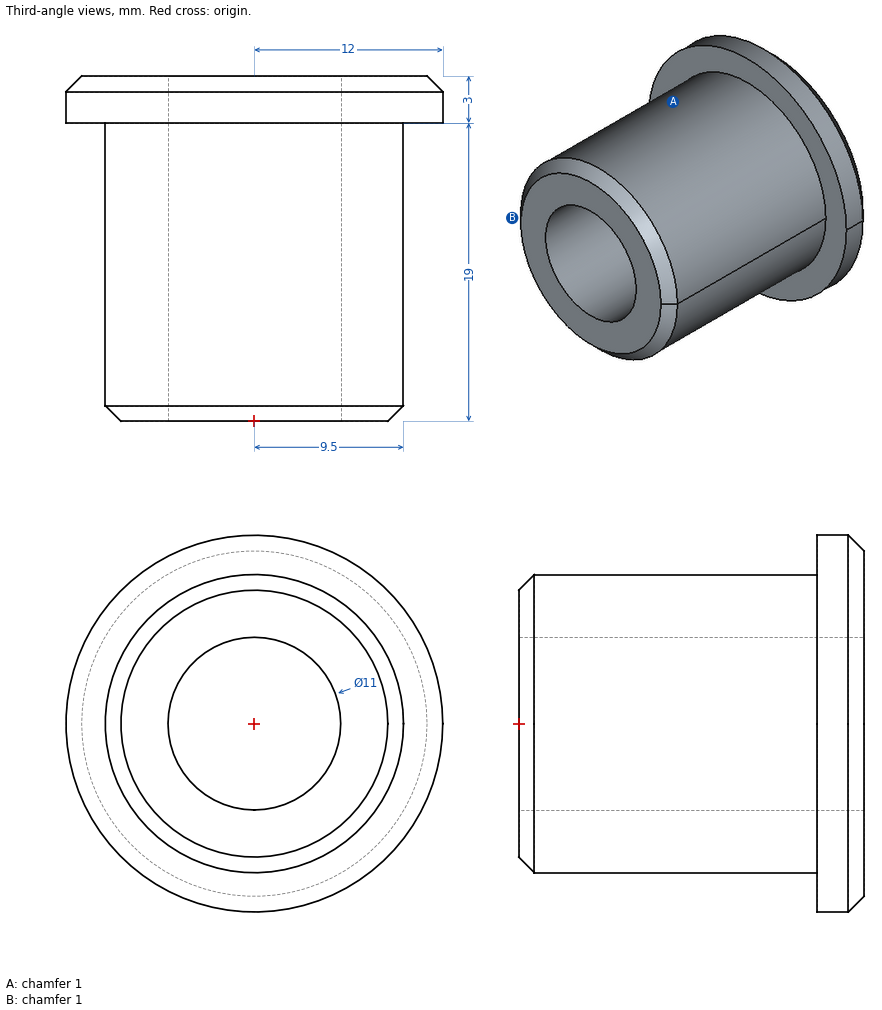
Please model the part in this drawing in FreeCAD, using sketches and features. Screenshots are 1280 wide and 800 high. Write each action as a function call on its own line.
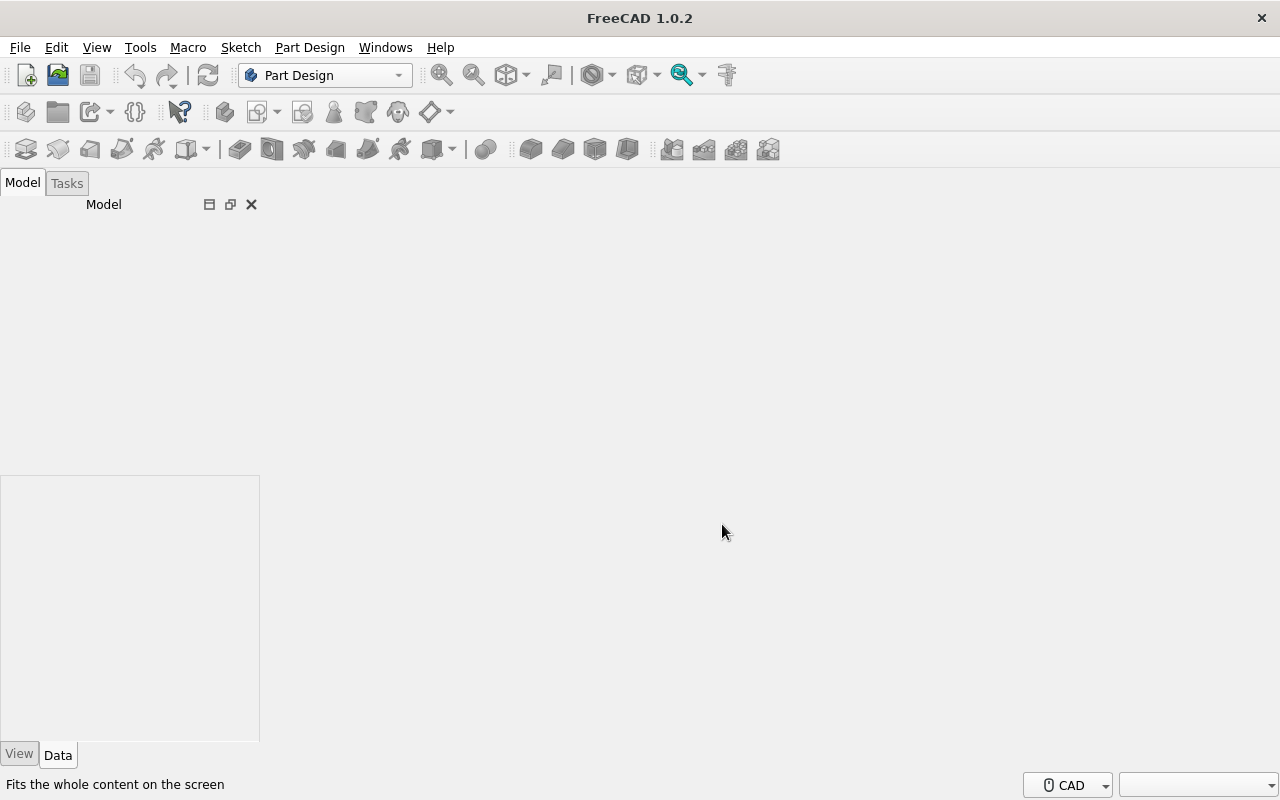
click(26, 76)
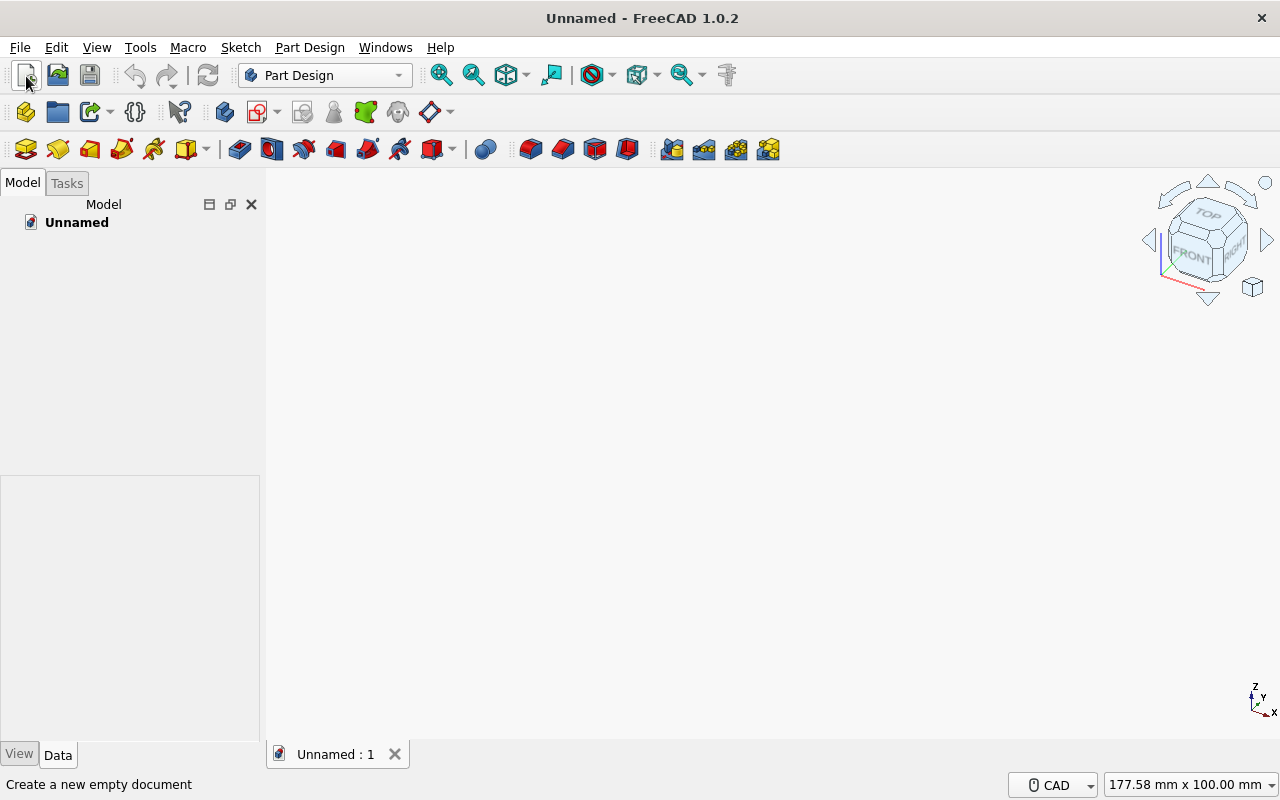
click(258, 112)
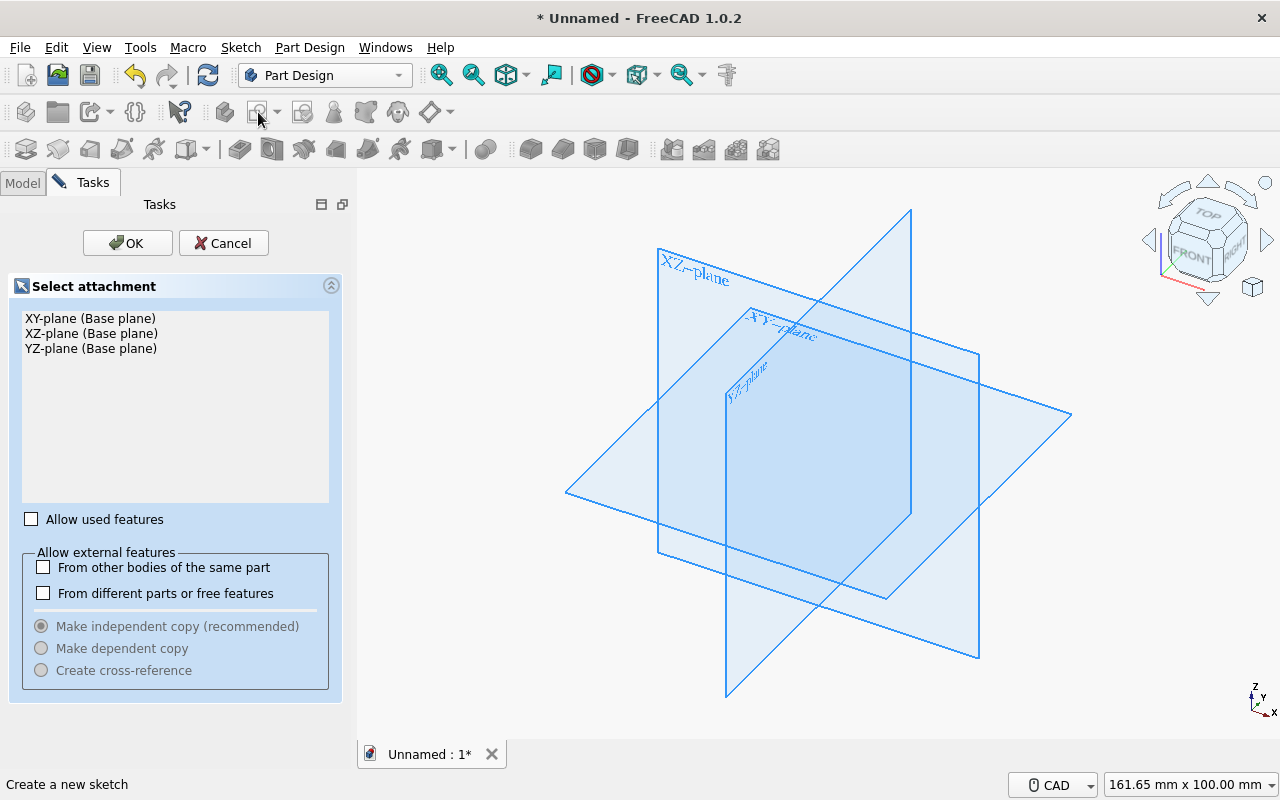
click(82, 318)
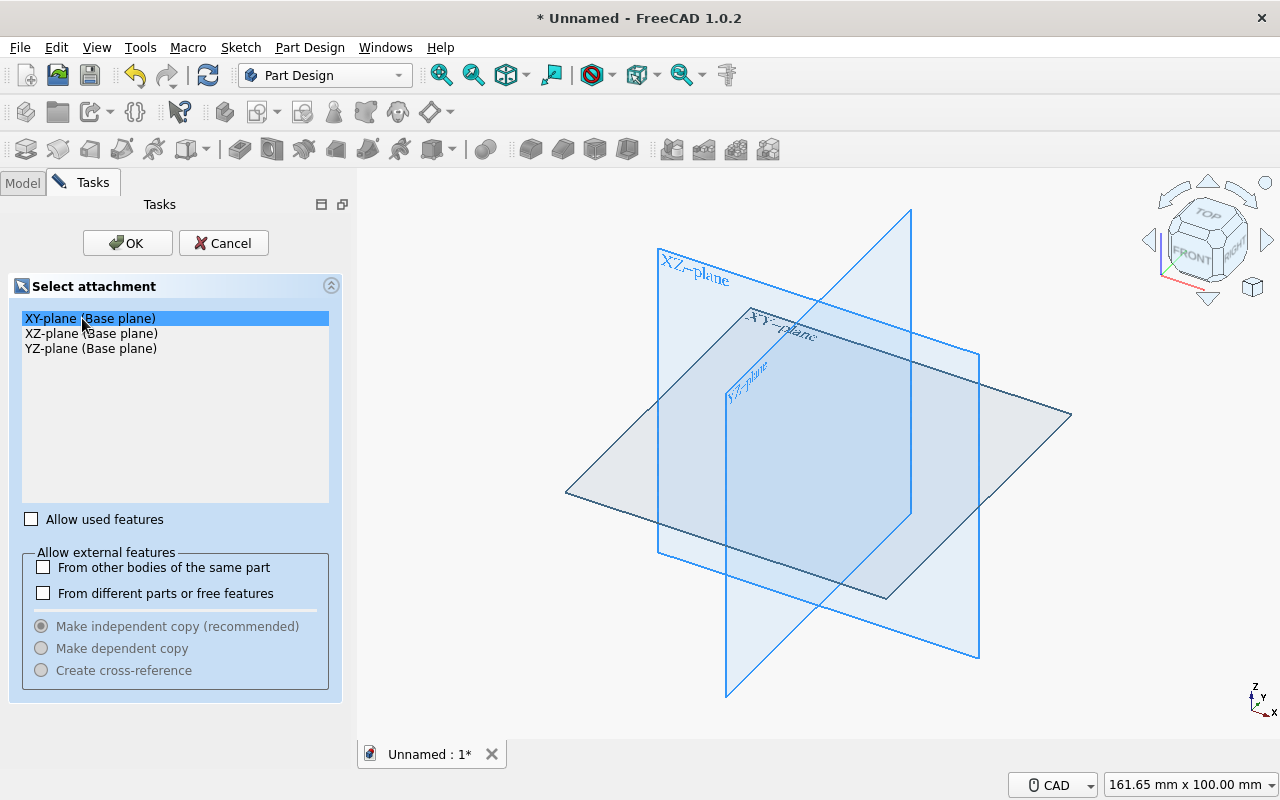
click(128, 243)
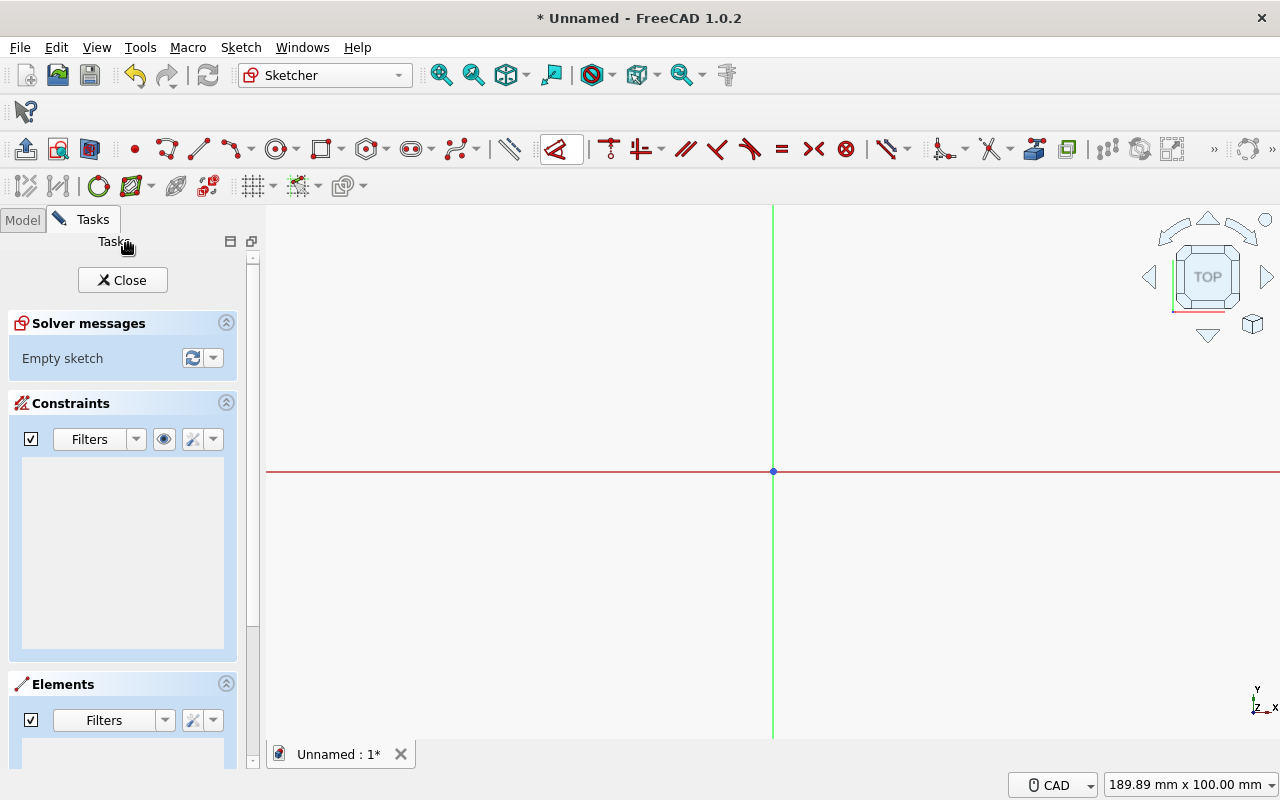
scroll(864, 379, up, 5)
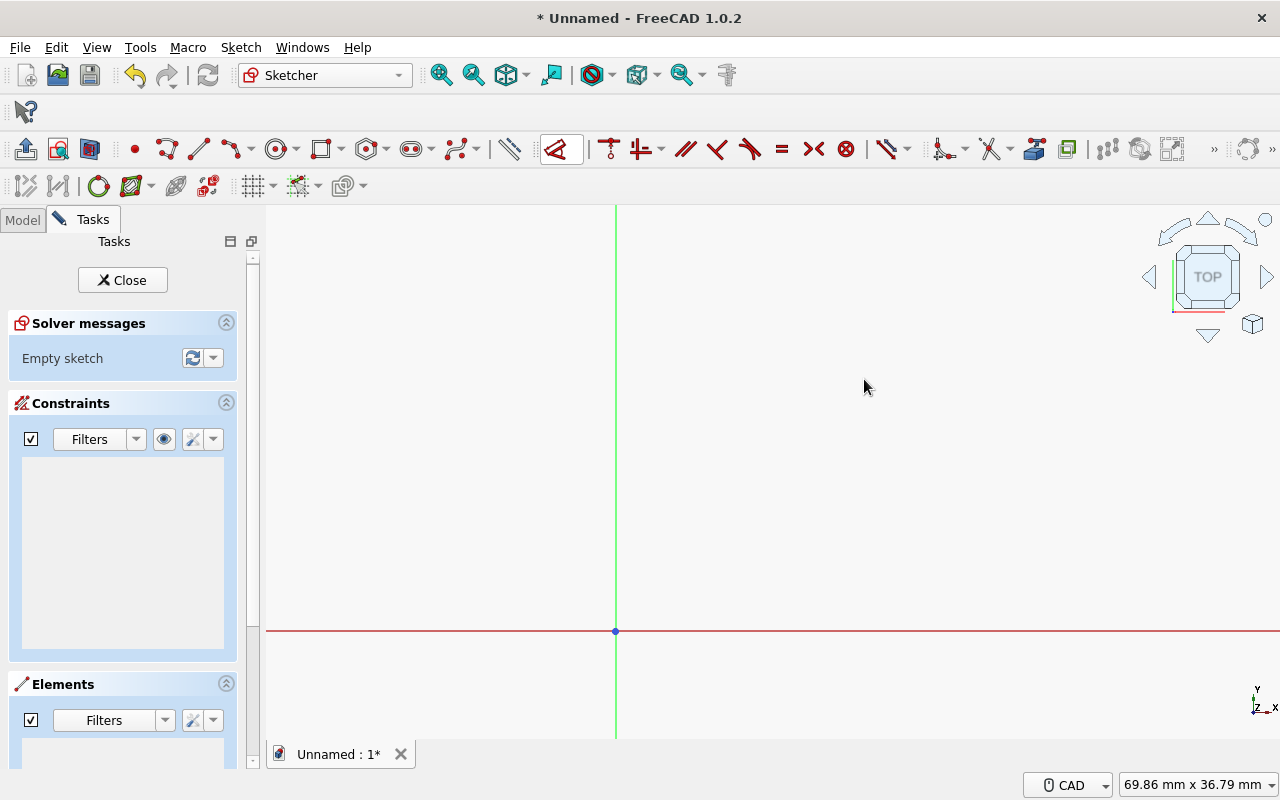
click(168, 150)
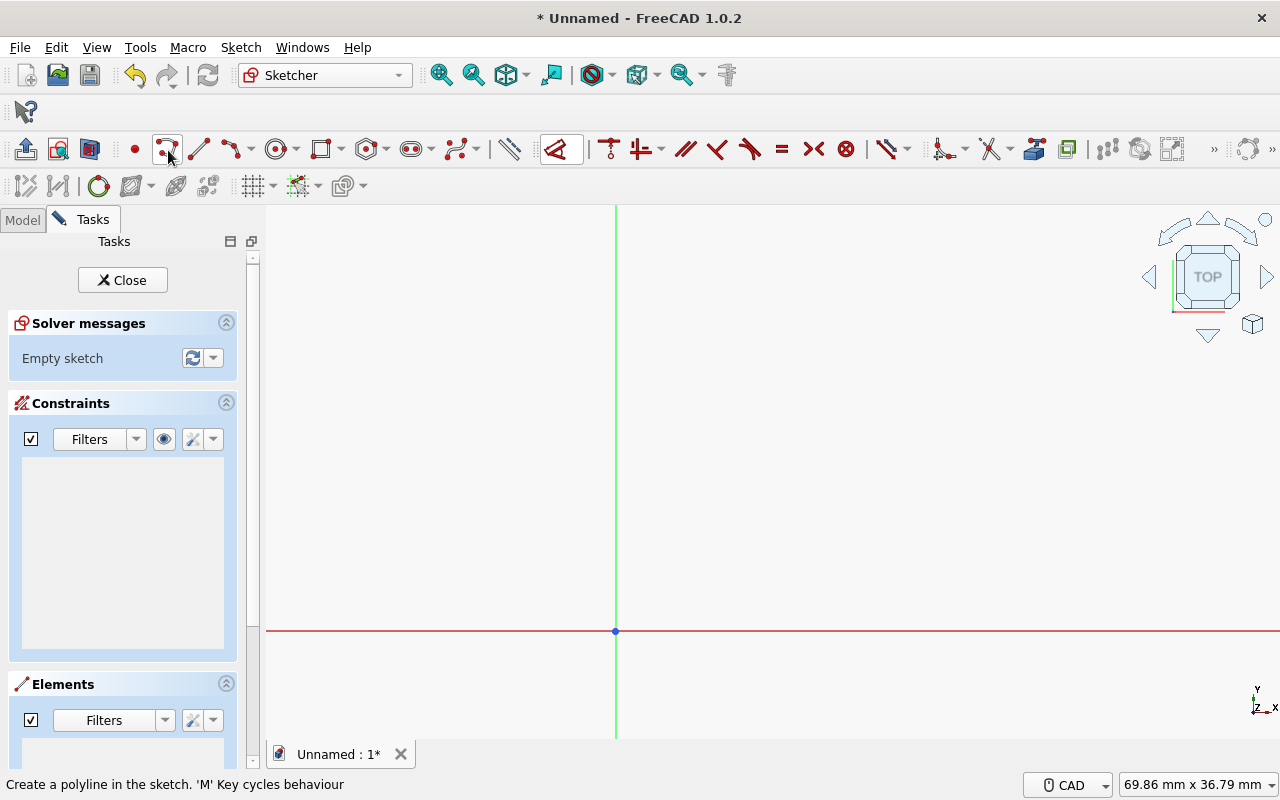
click(616, 631)
click(754, 622)
click(754, 355)
click(790, 355)
click(790, 312)
click(625, 312)
click(616, 631)
key(Escape)
key(Escape)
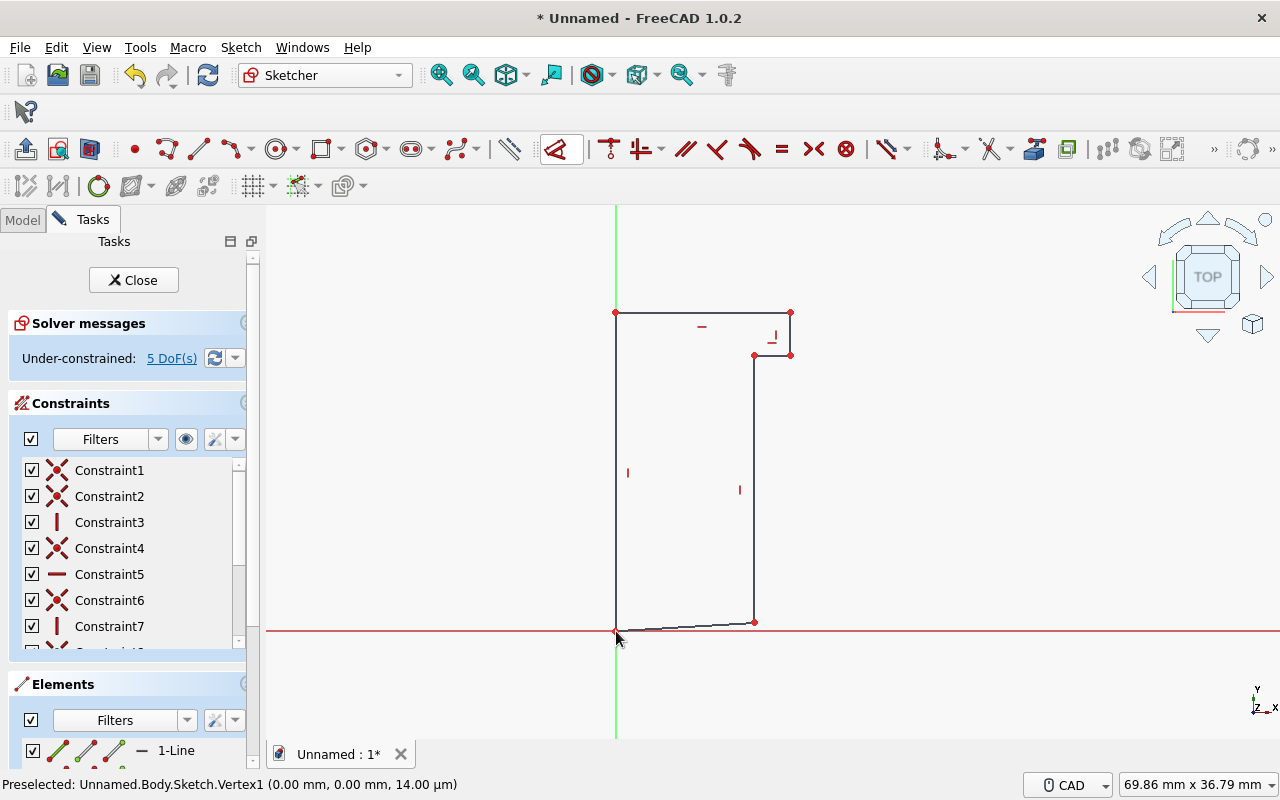
click(657, 629)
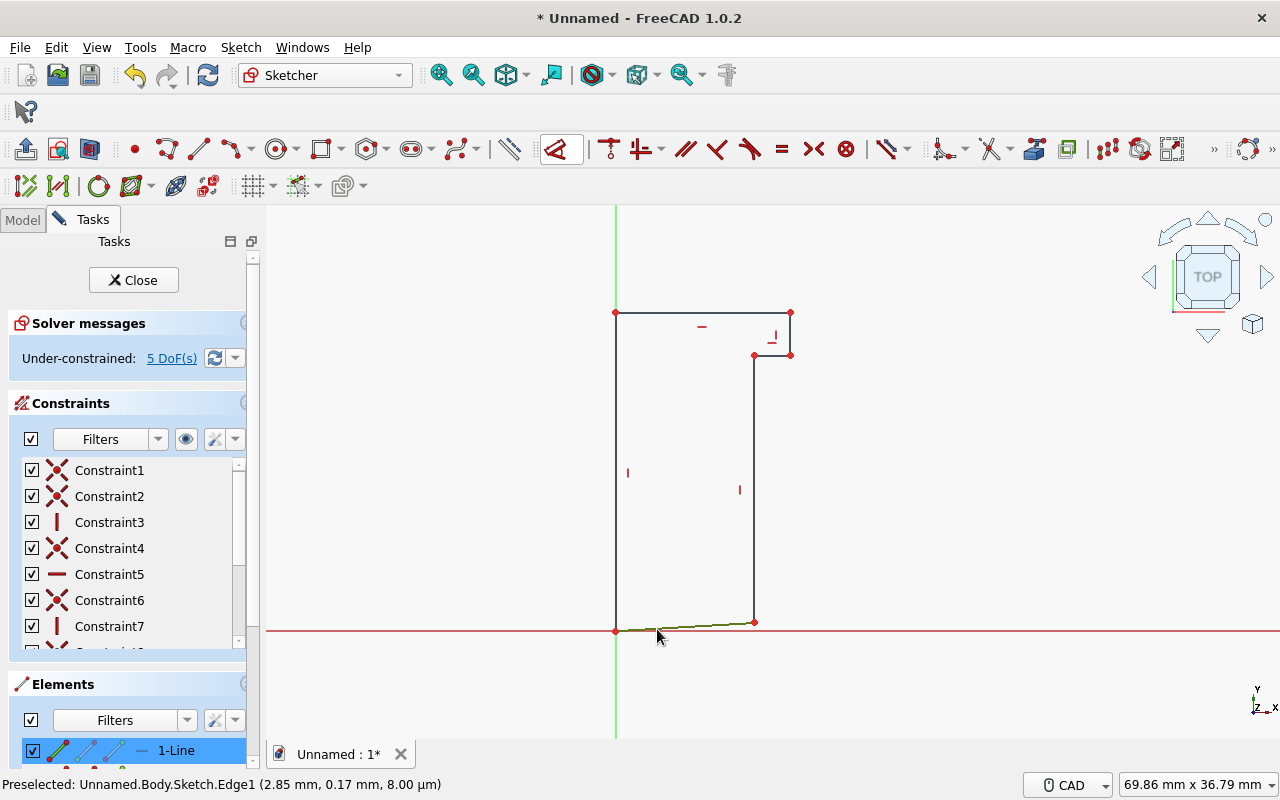
key(h)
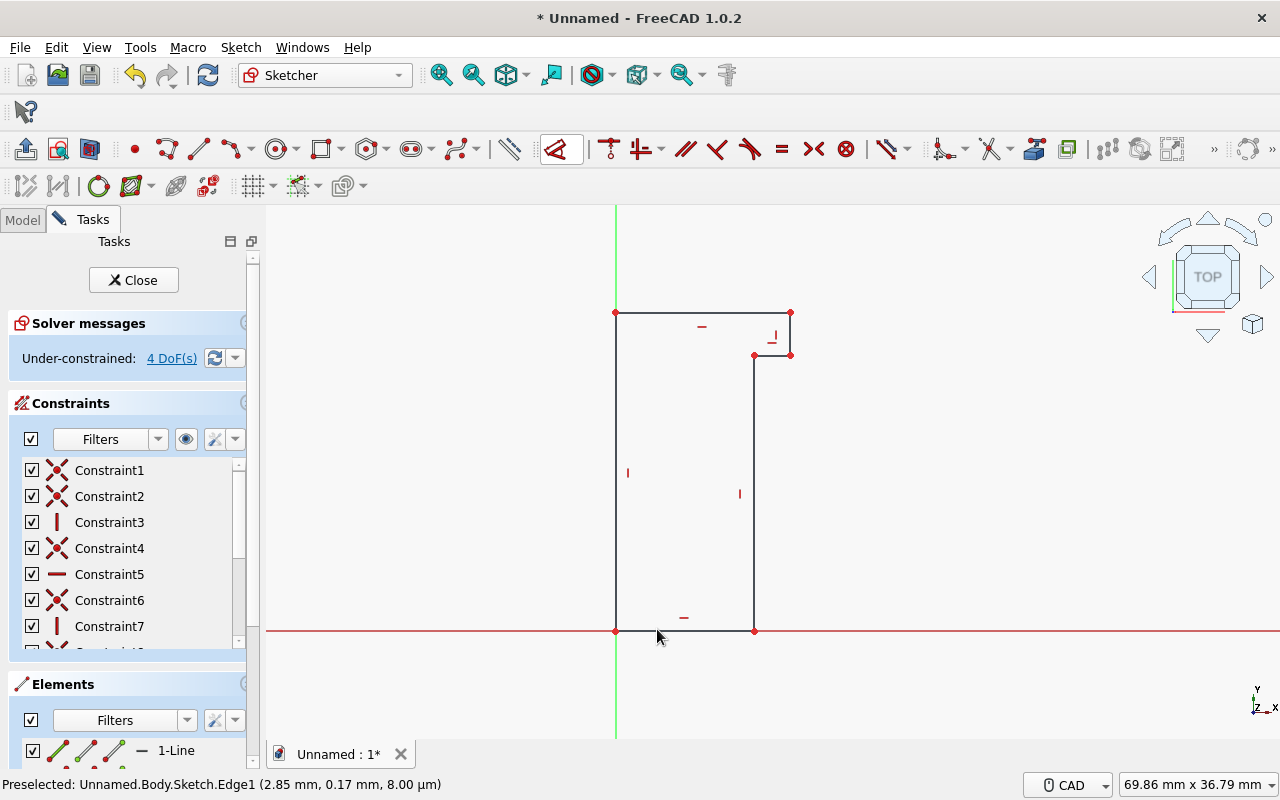
click(790, 343)